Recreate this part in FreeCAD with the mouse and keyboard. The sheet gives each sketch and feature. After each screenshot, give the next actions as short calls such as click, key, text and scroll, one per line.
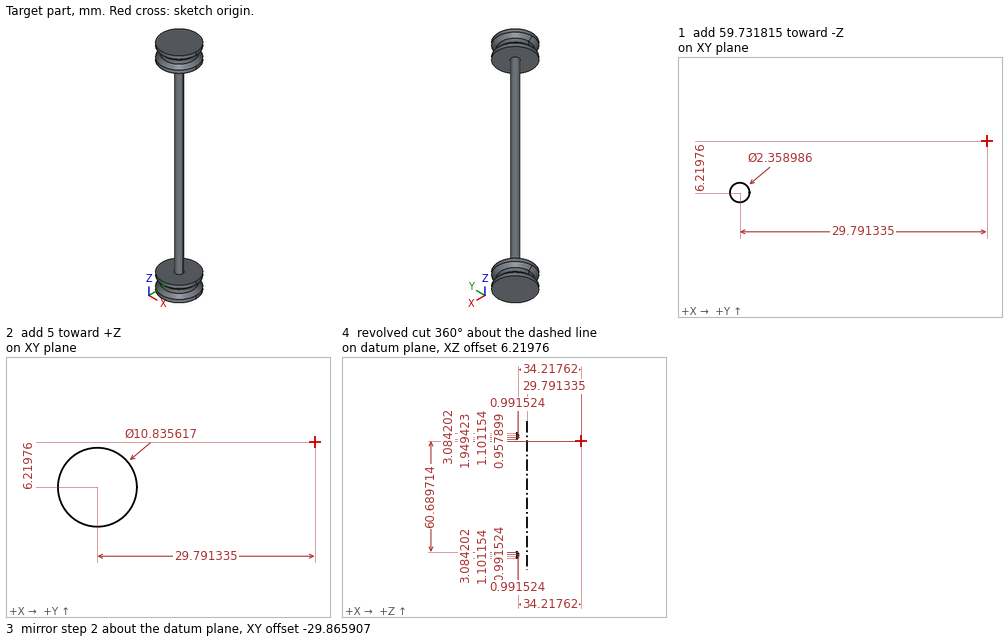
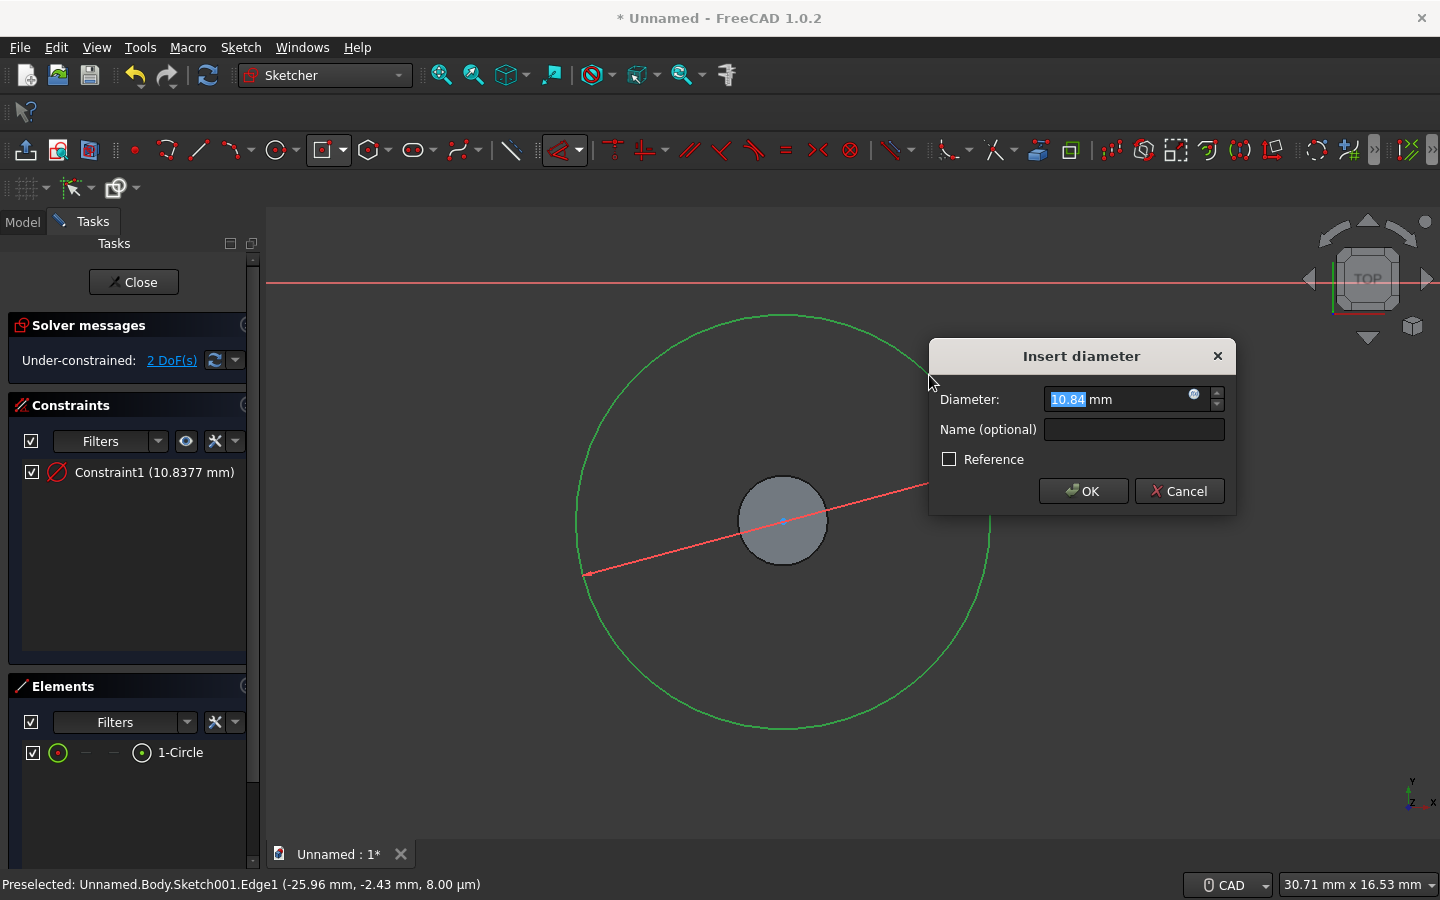
text(10.835617)
key(Return)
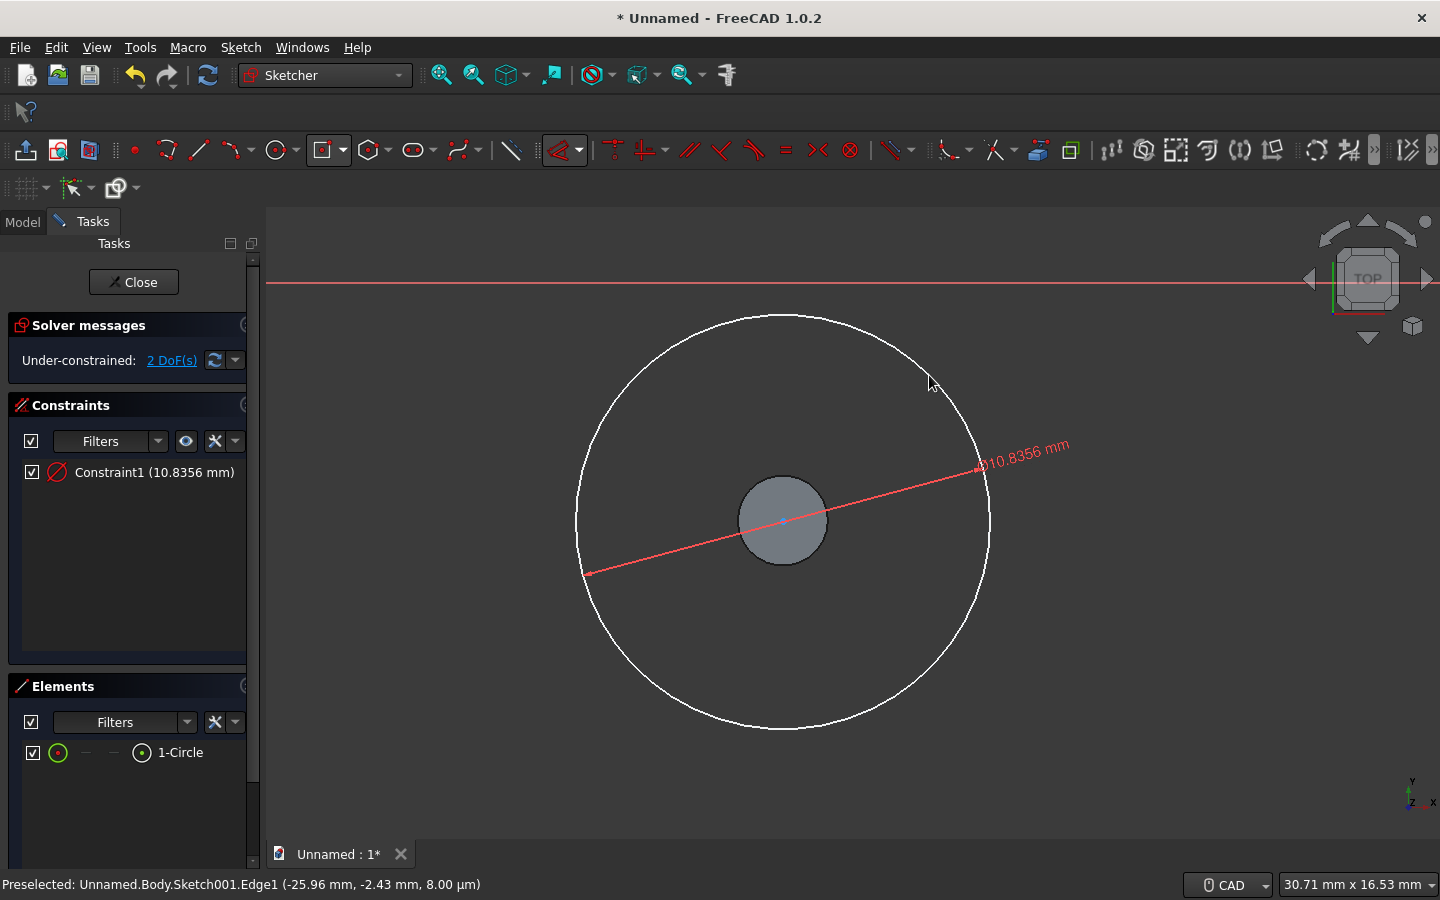
click(783, 522)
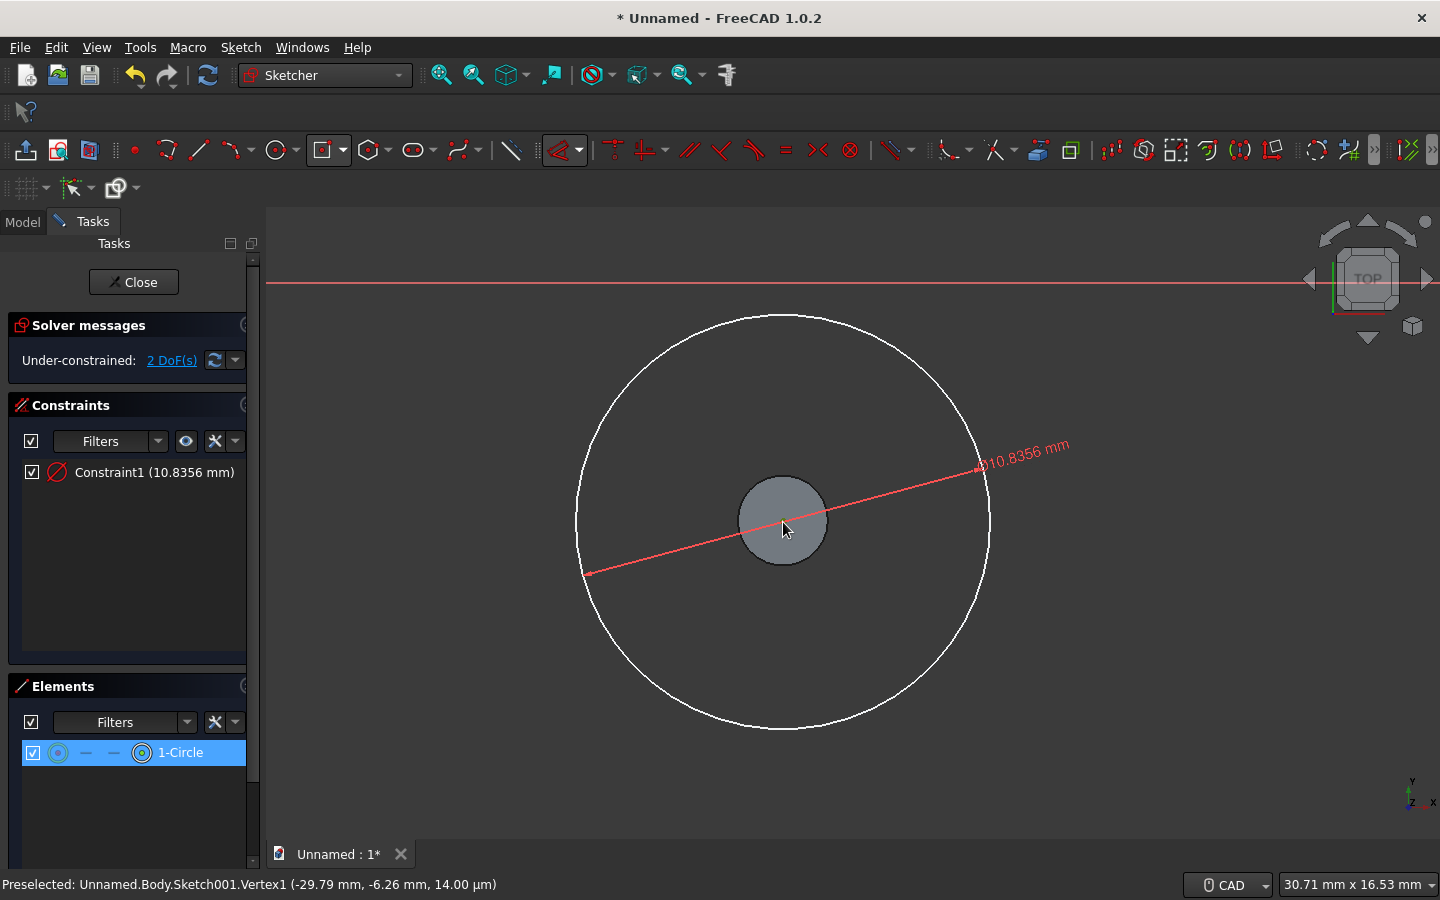
key(i)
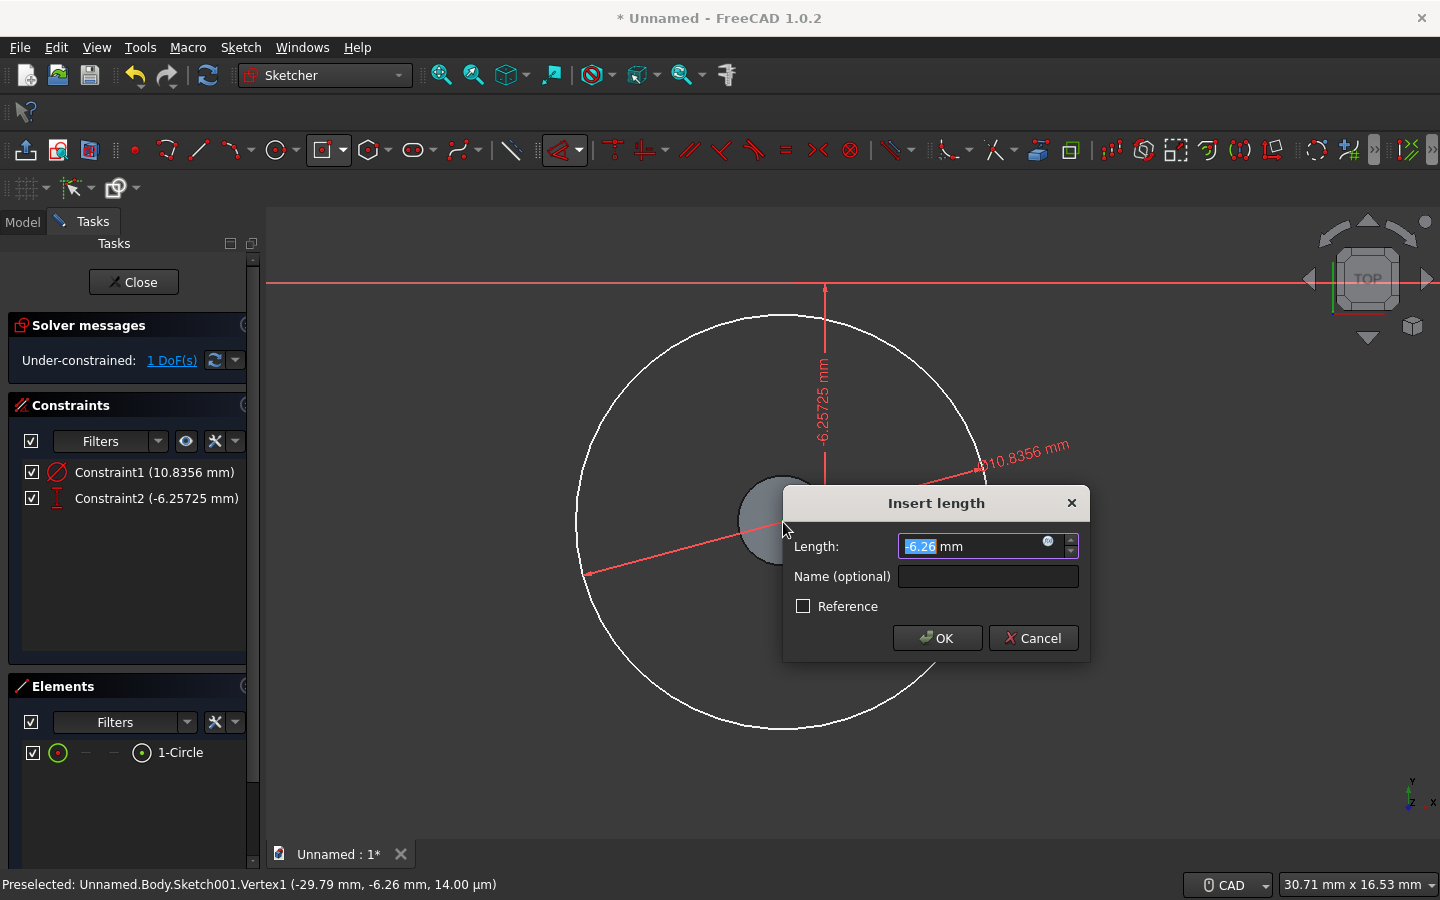
text(-6.21976)
key(Return)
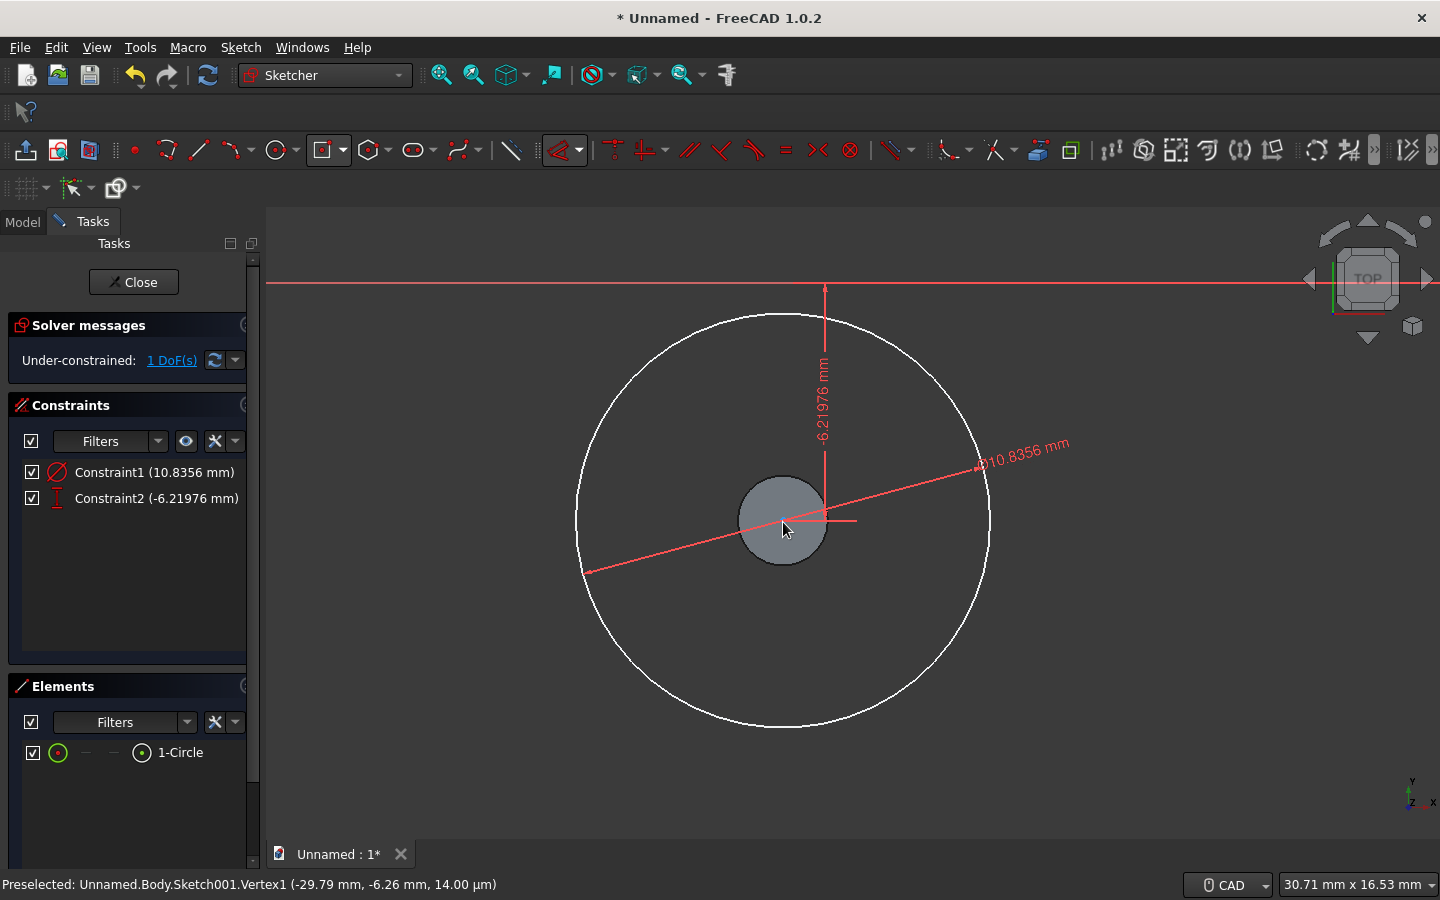
click(783, 521)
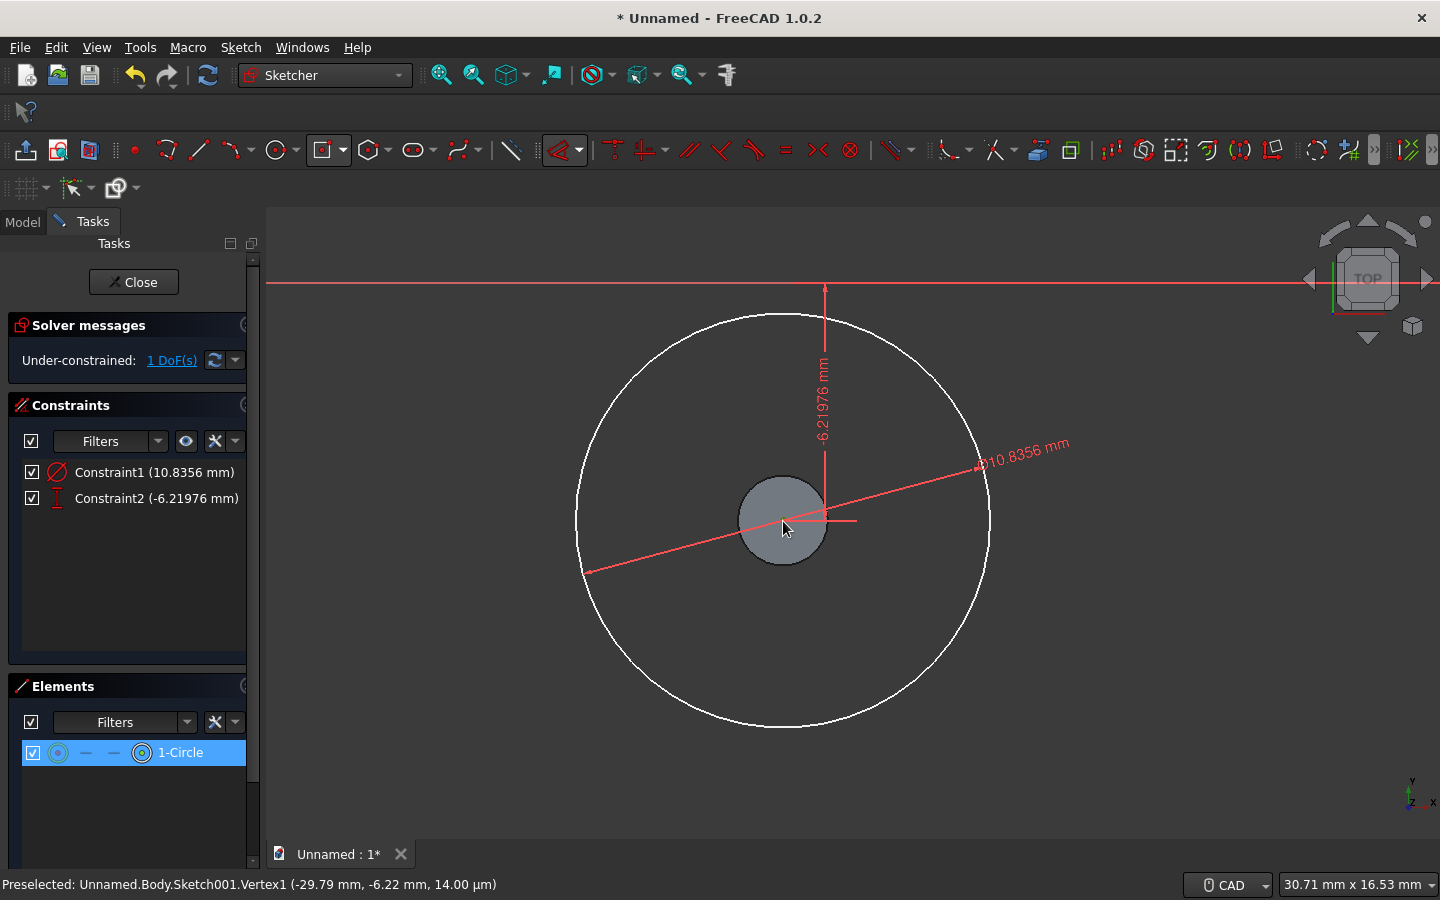
key(l)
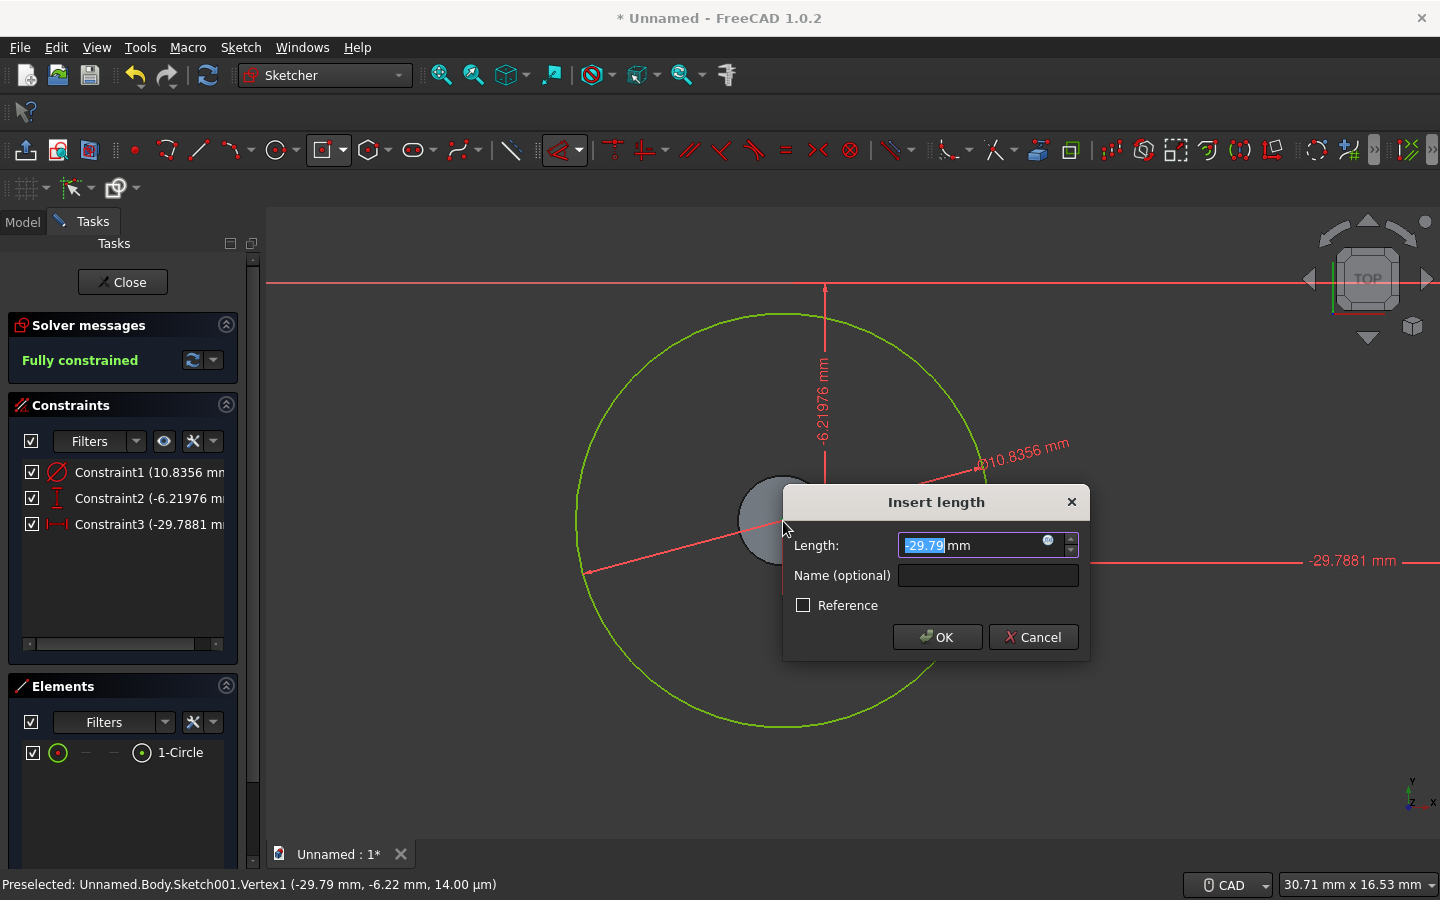
text(-29.791335)
key(Return)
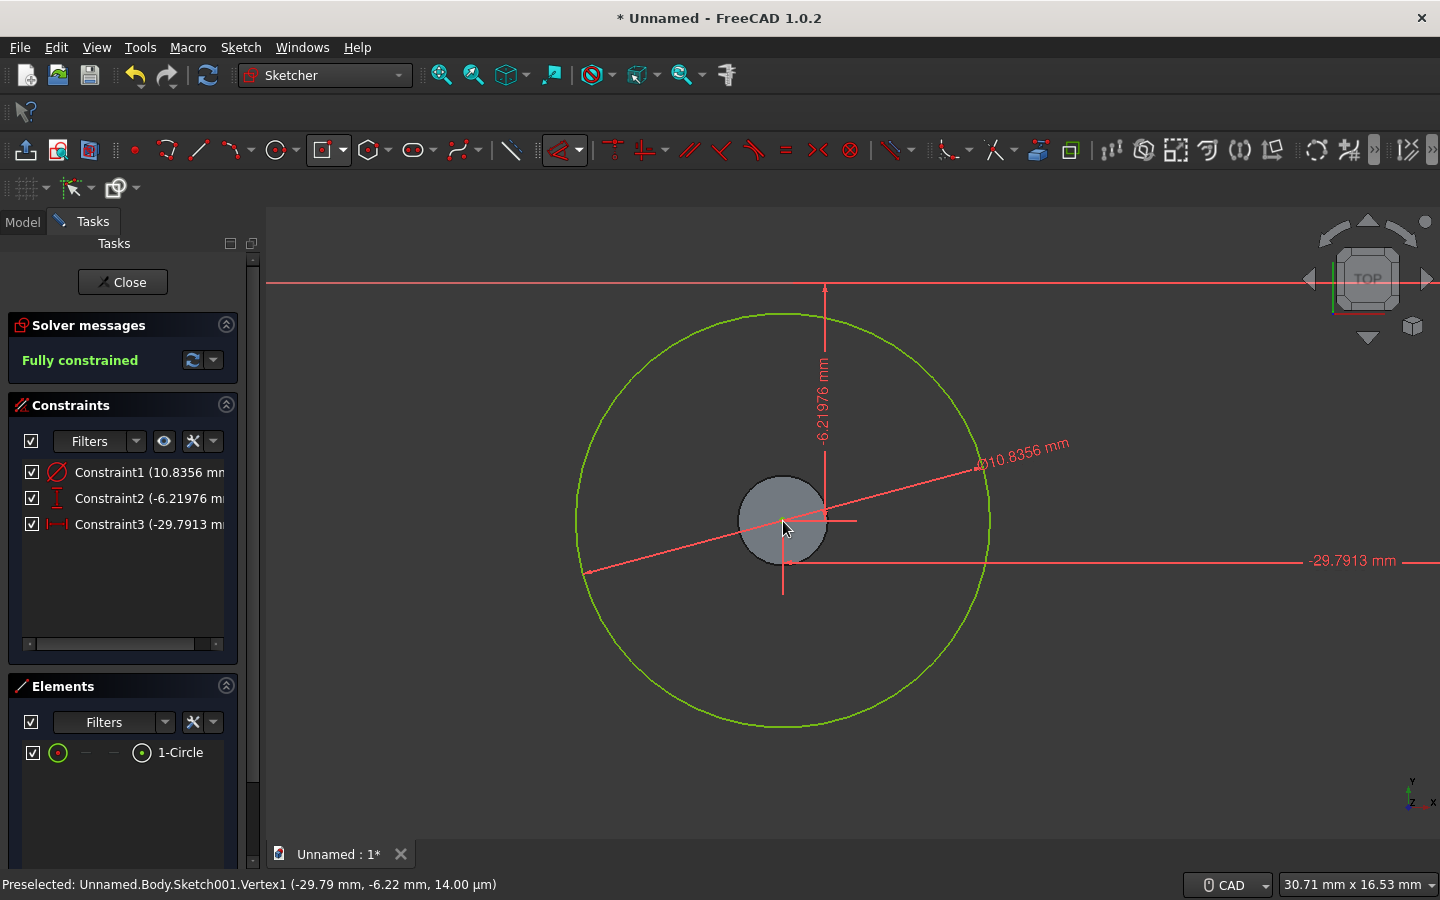
click(123, 282)